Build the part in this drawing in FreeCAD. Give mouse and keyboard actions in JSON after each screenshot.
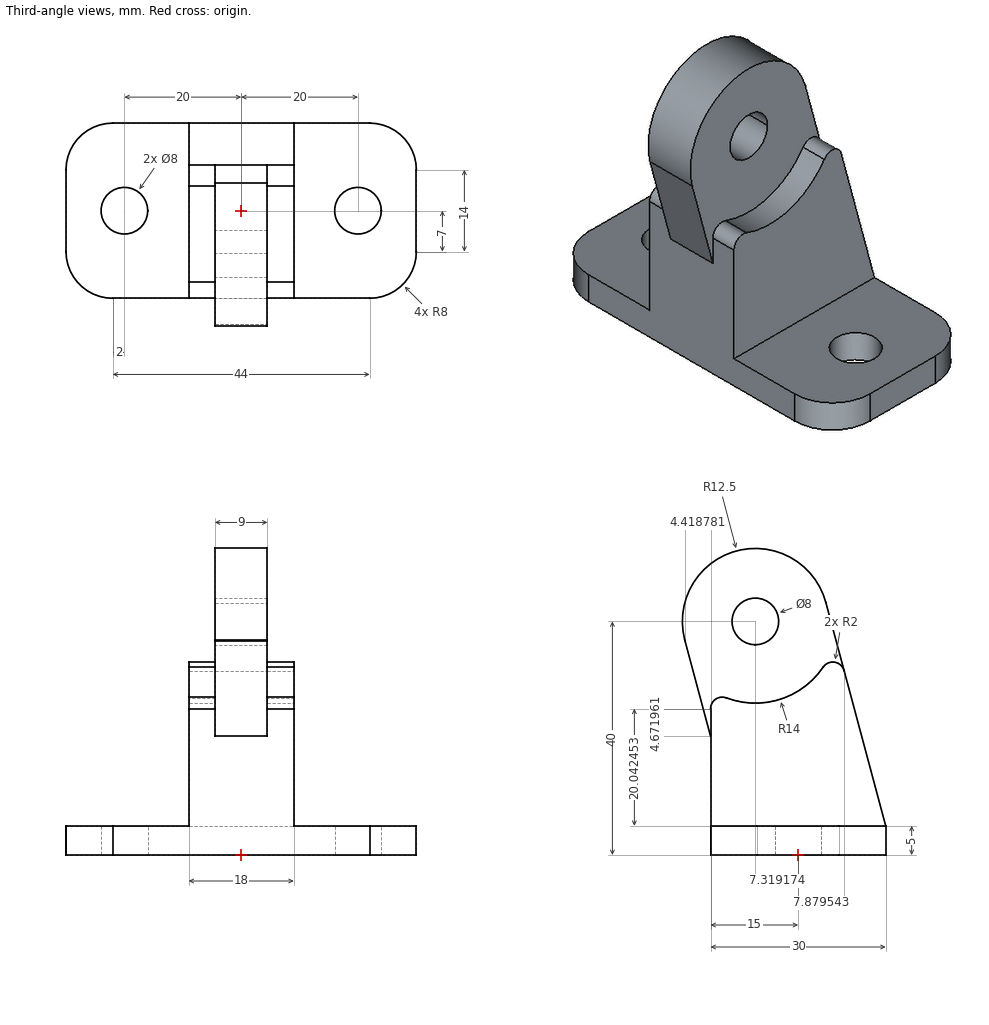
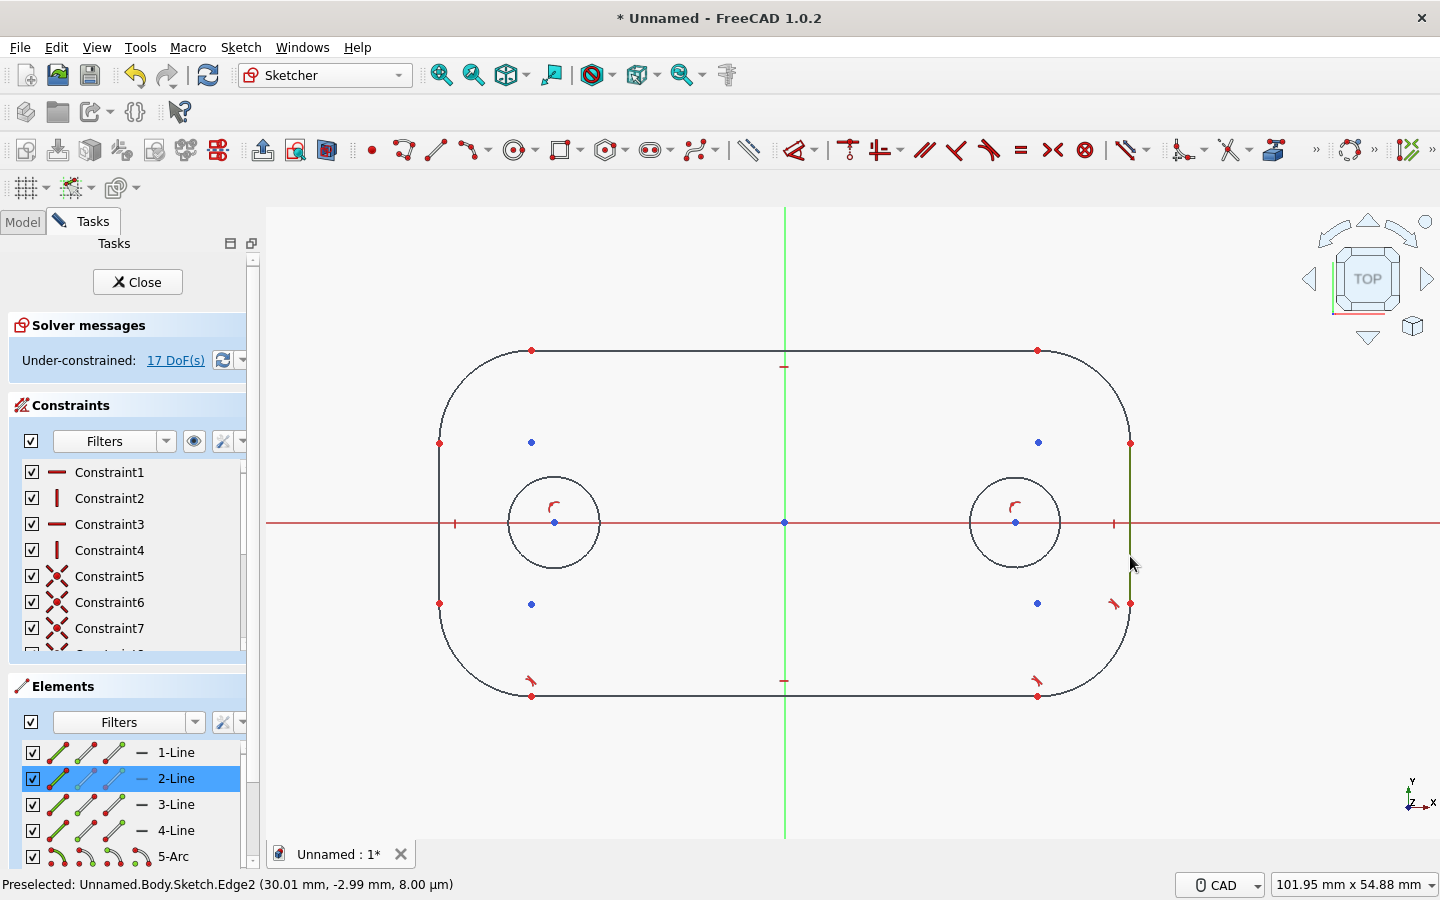
{"action": "left_click", "coordinate": [1120, 401]}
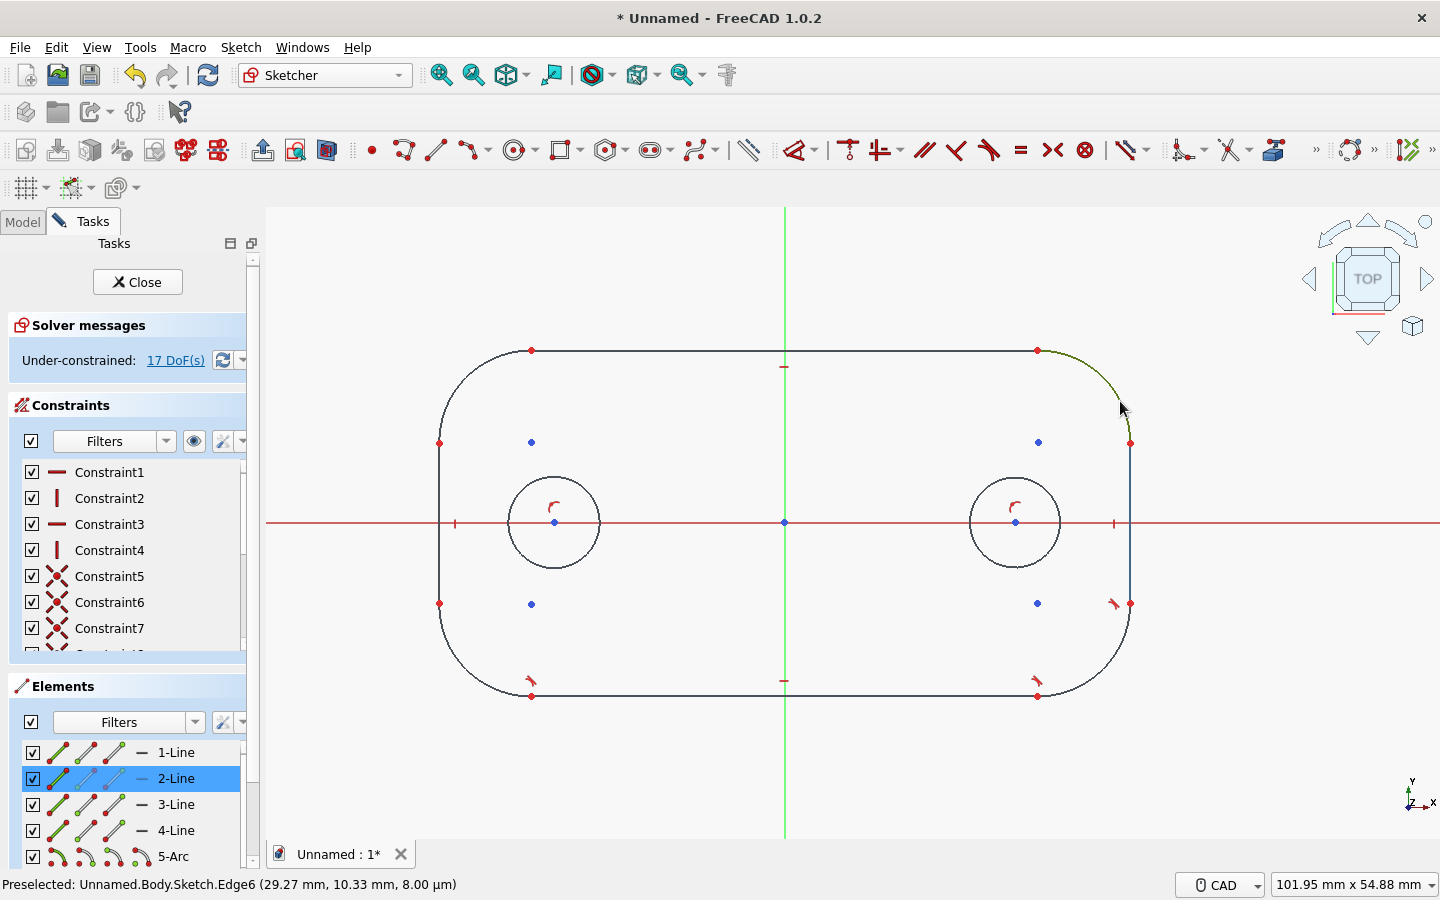
{"action": "key", "text": "t"}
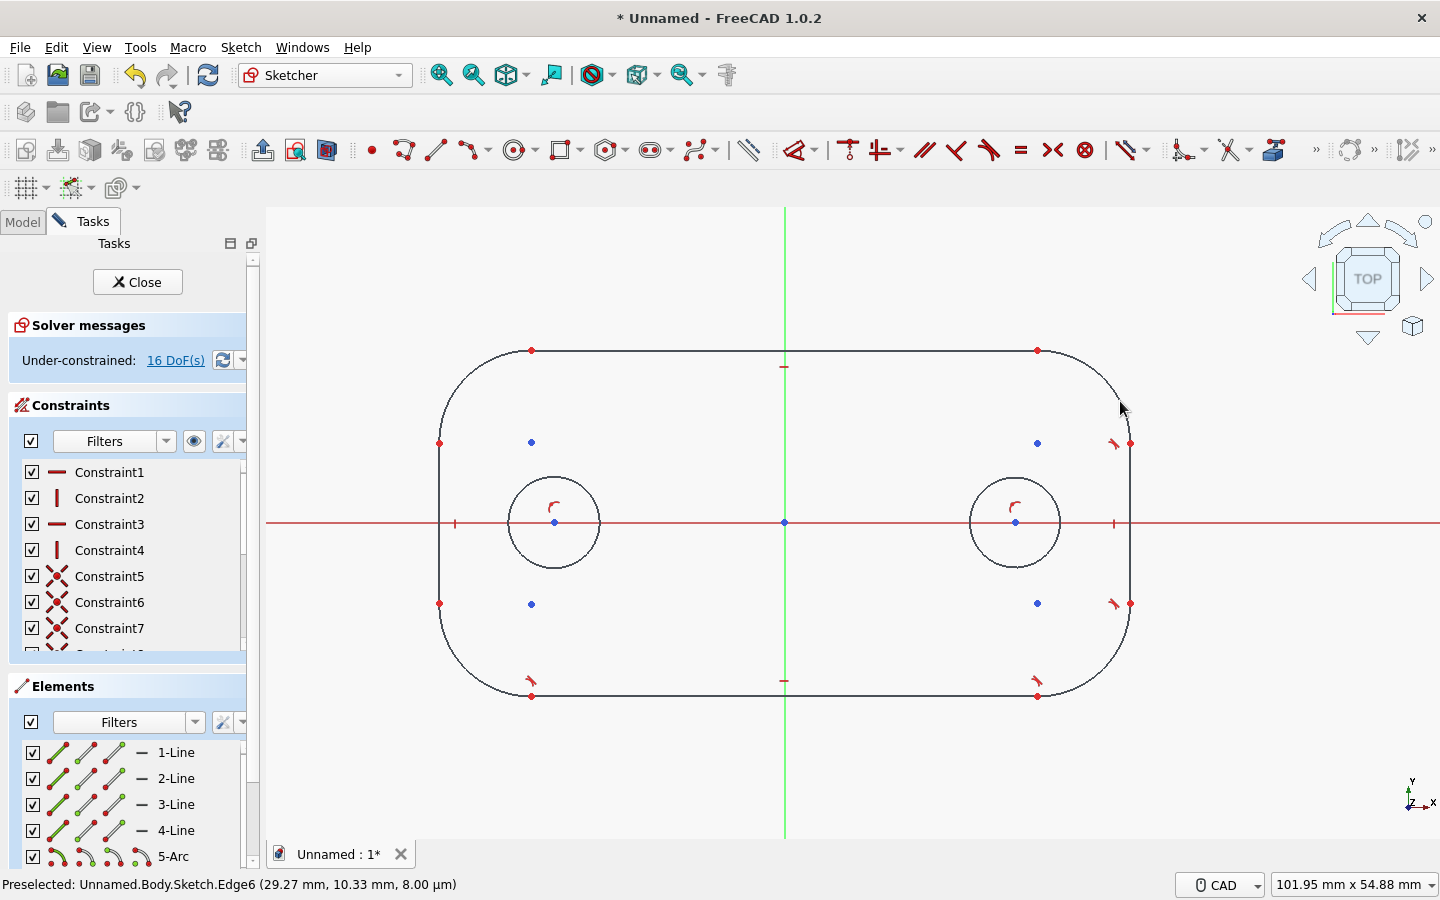
{"action": "left_click", "coordinate": [885, 351]}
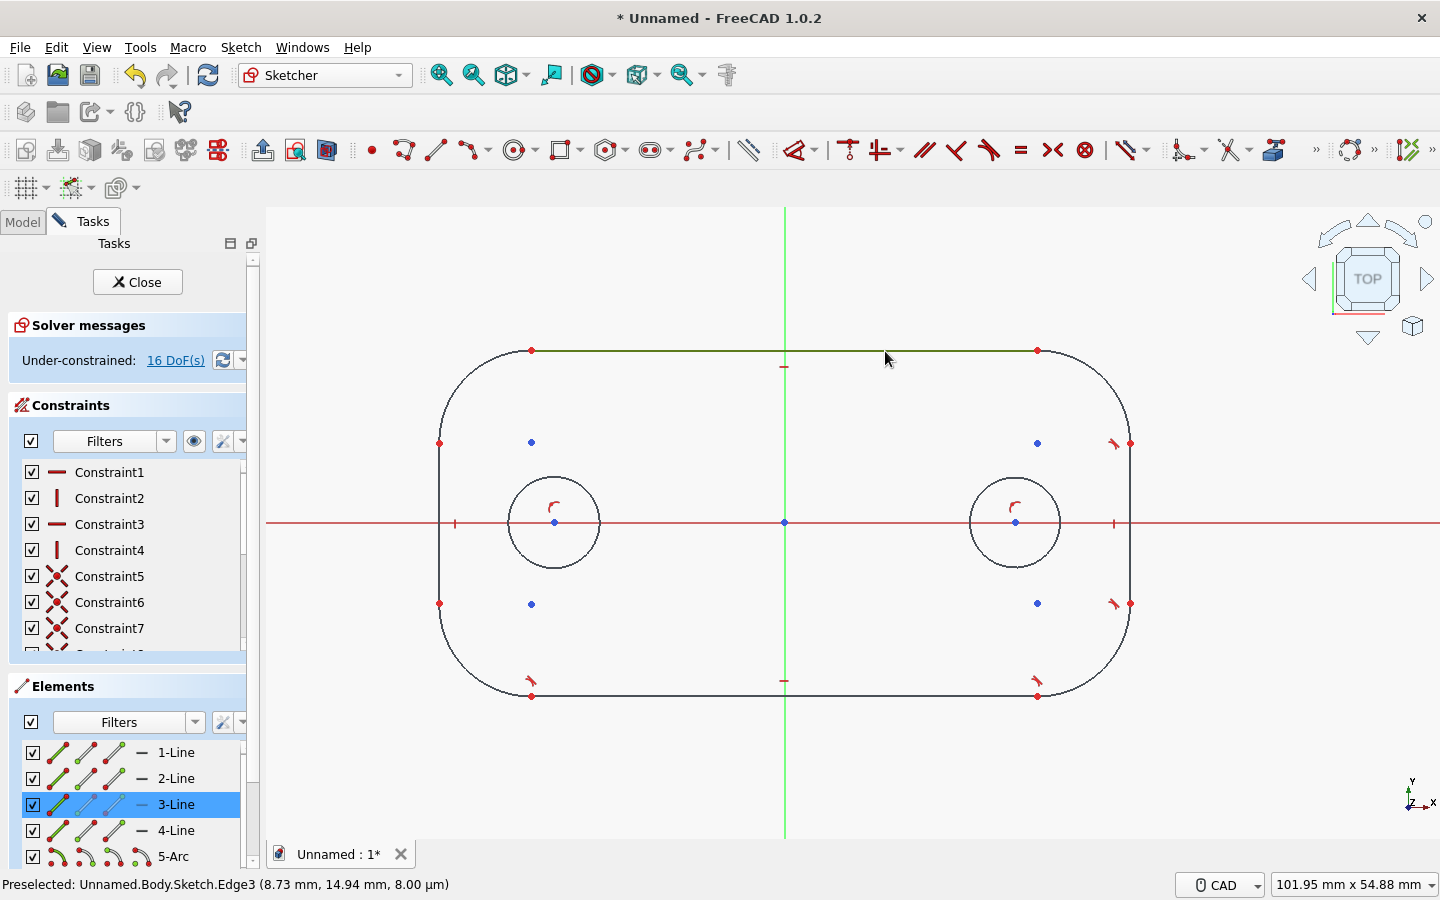
{"action": "left_click", "coordinate": [1120, 401]}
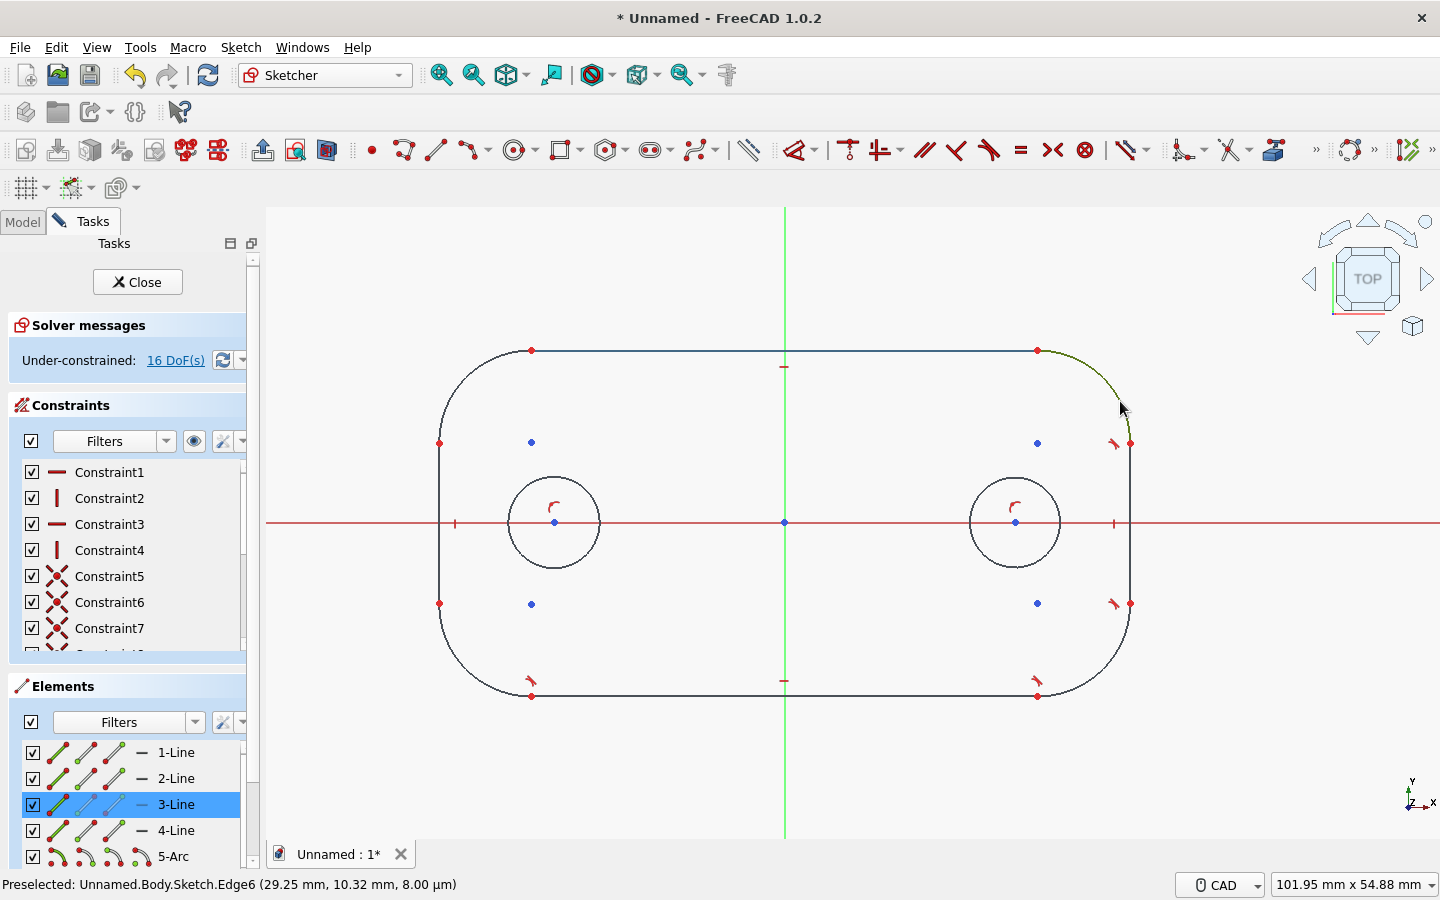
{"action": "key", "text": "t"}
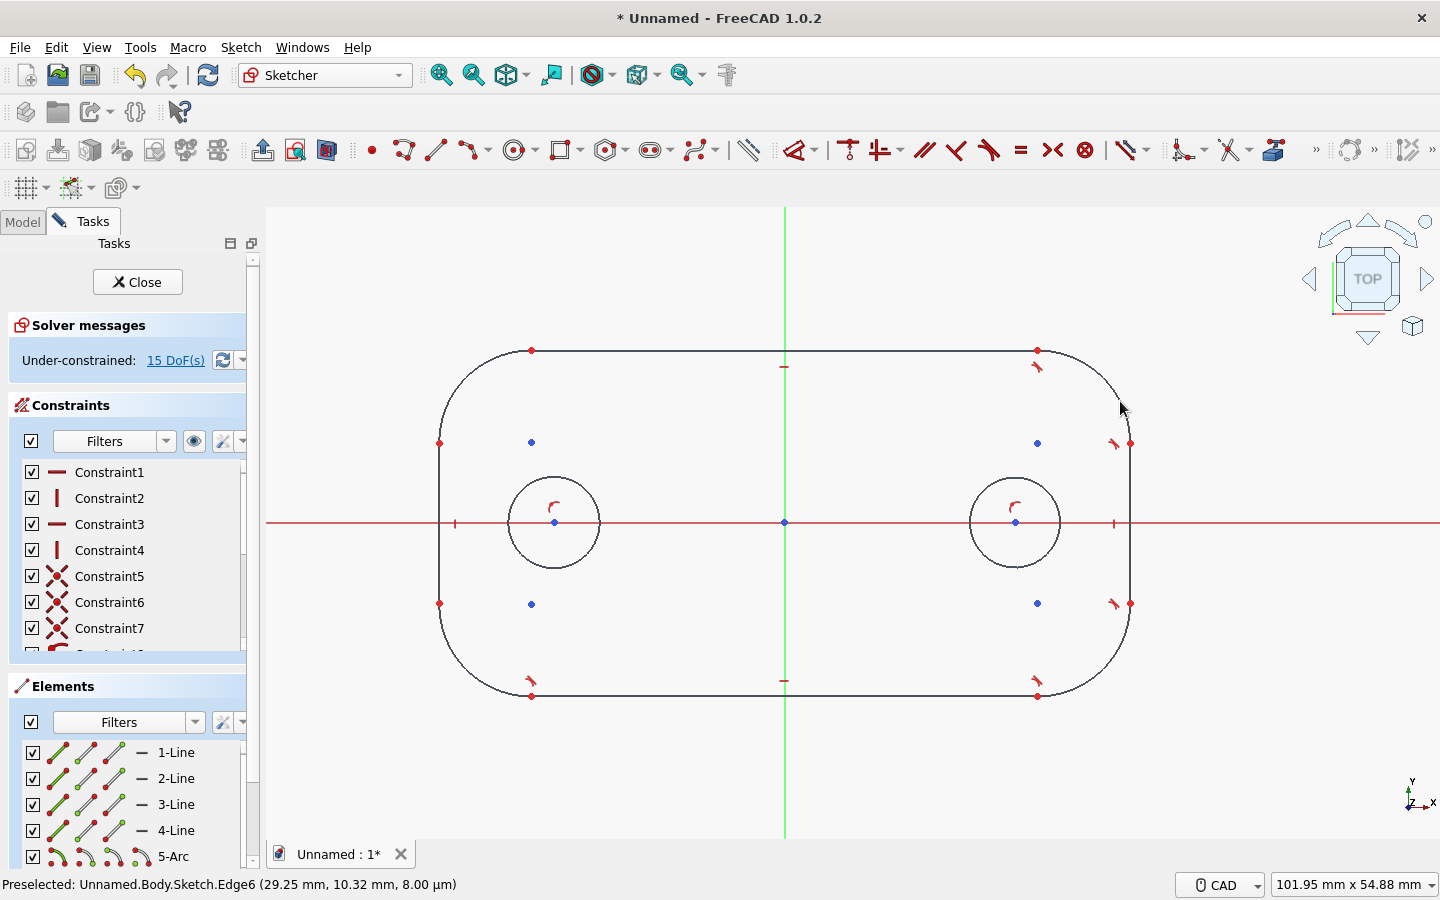
{"action": "left_click", "coordinate": [885, 351]}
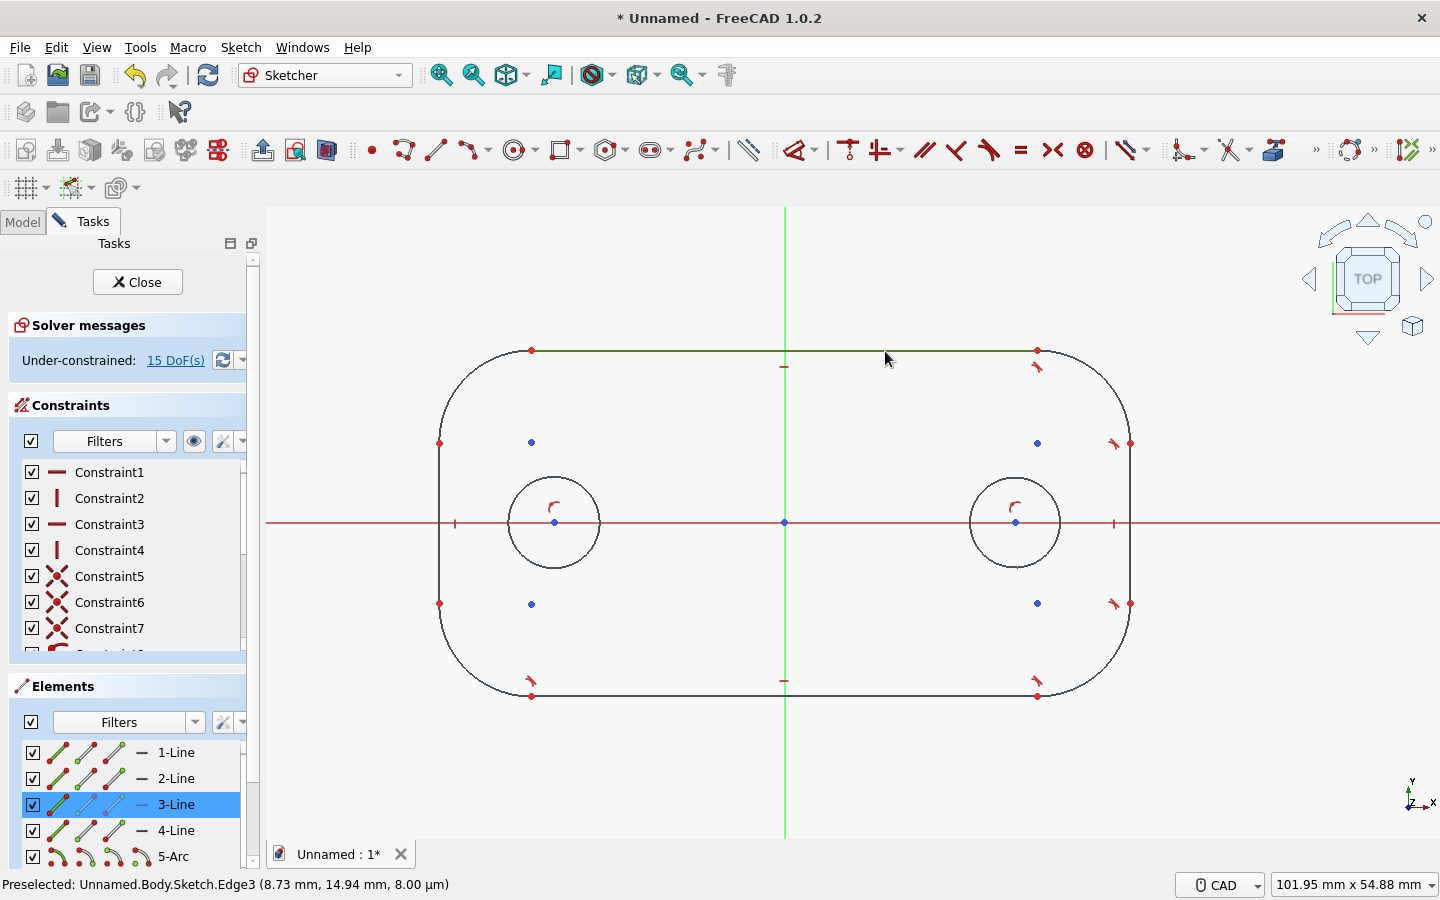
{"action": "left_click", "coordinate": [489, 361]}